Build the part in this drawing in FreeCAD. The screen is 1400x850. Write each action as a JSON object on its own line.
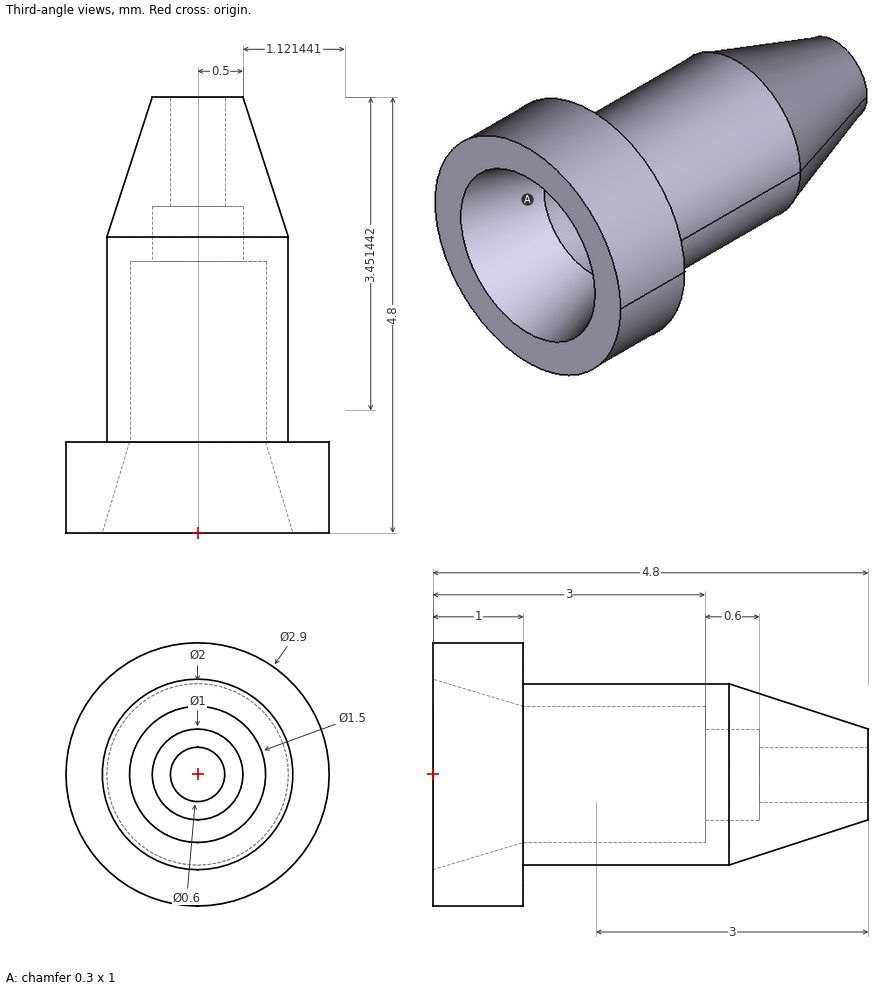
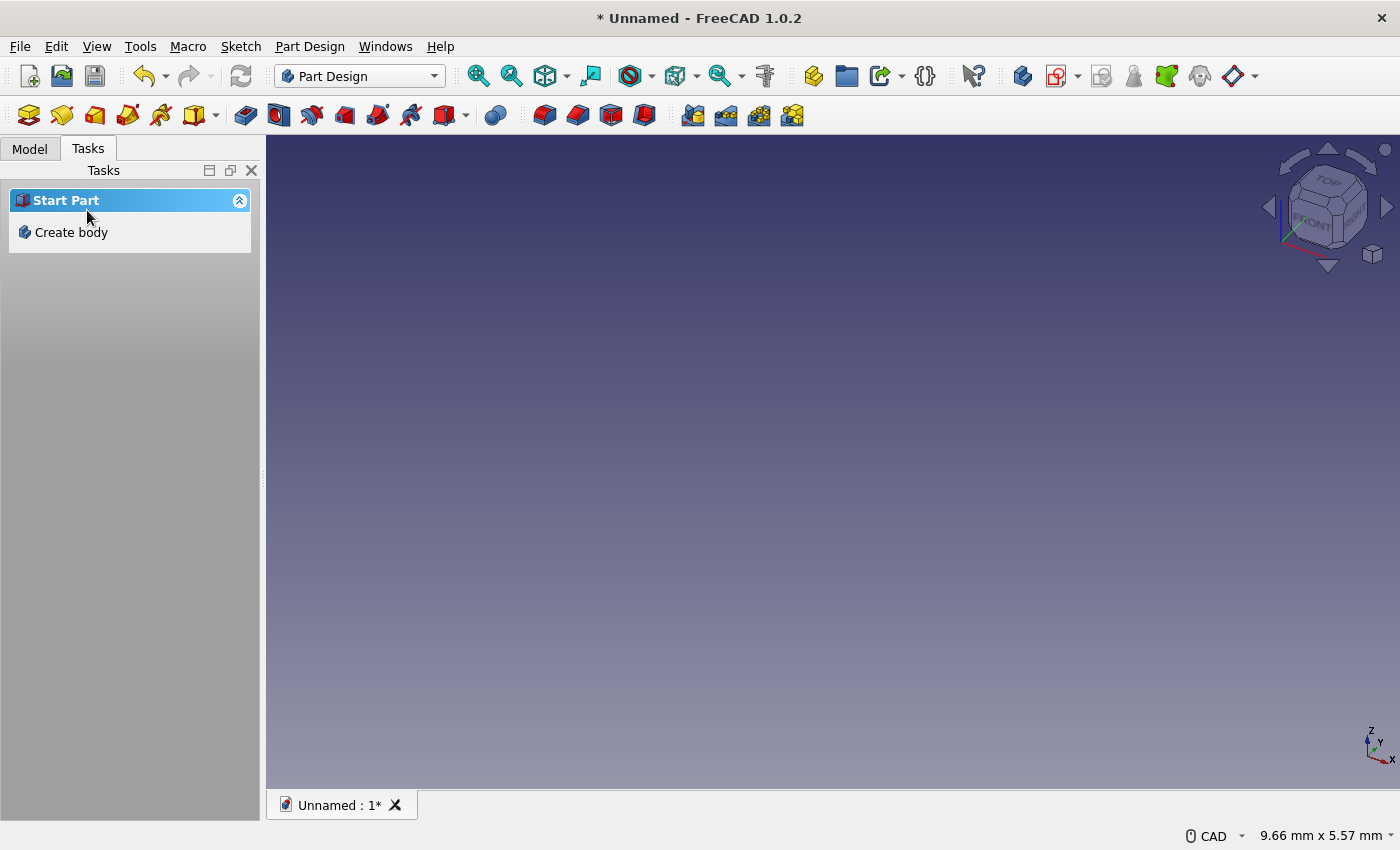
{"action": "left_click", "coordinate": [479, 76]}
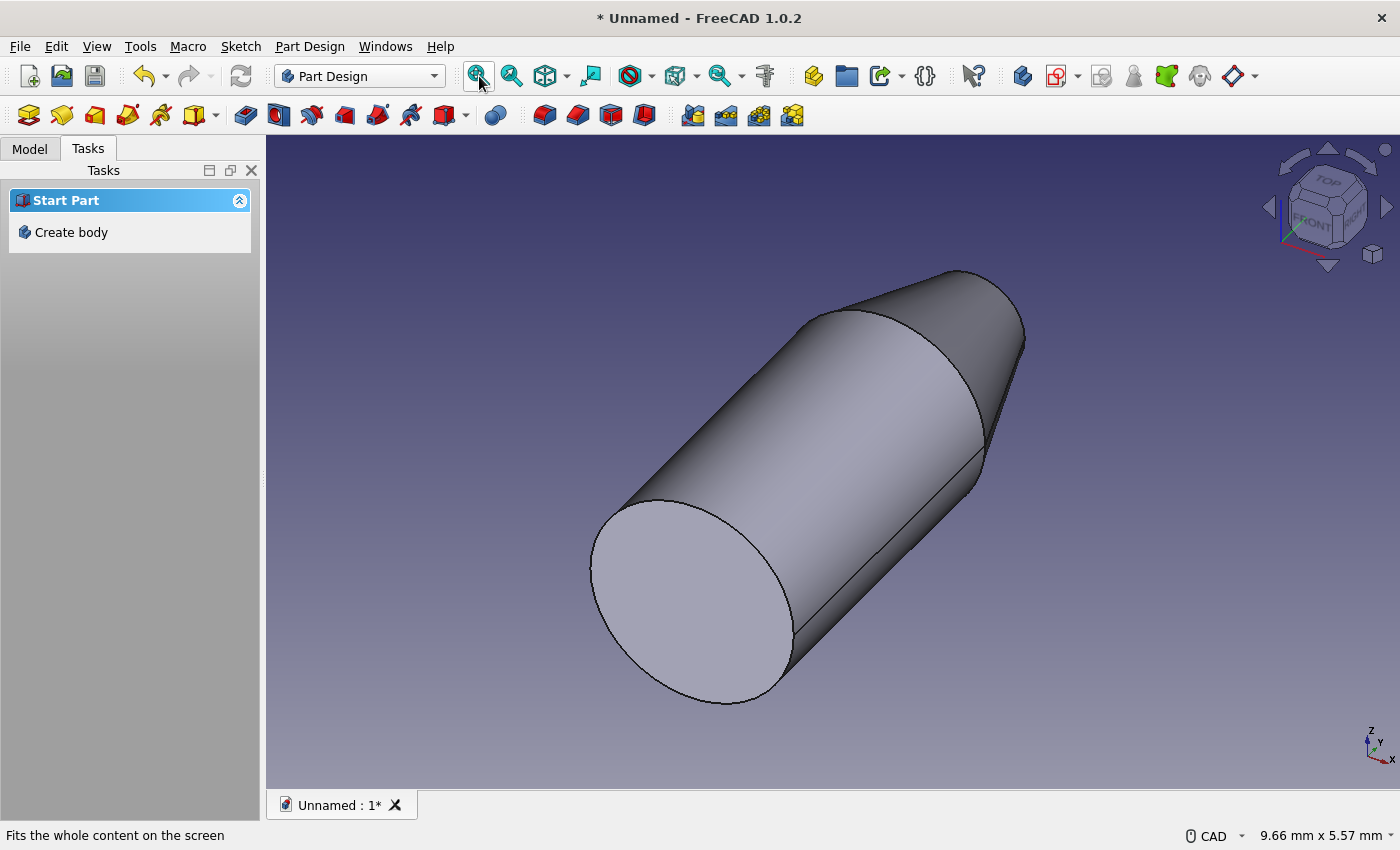
{"action": "left_click", "coordinate": [692, 601]}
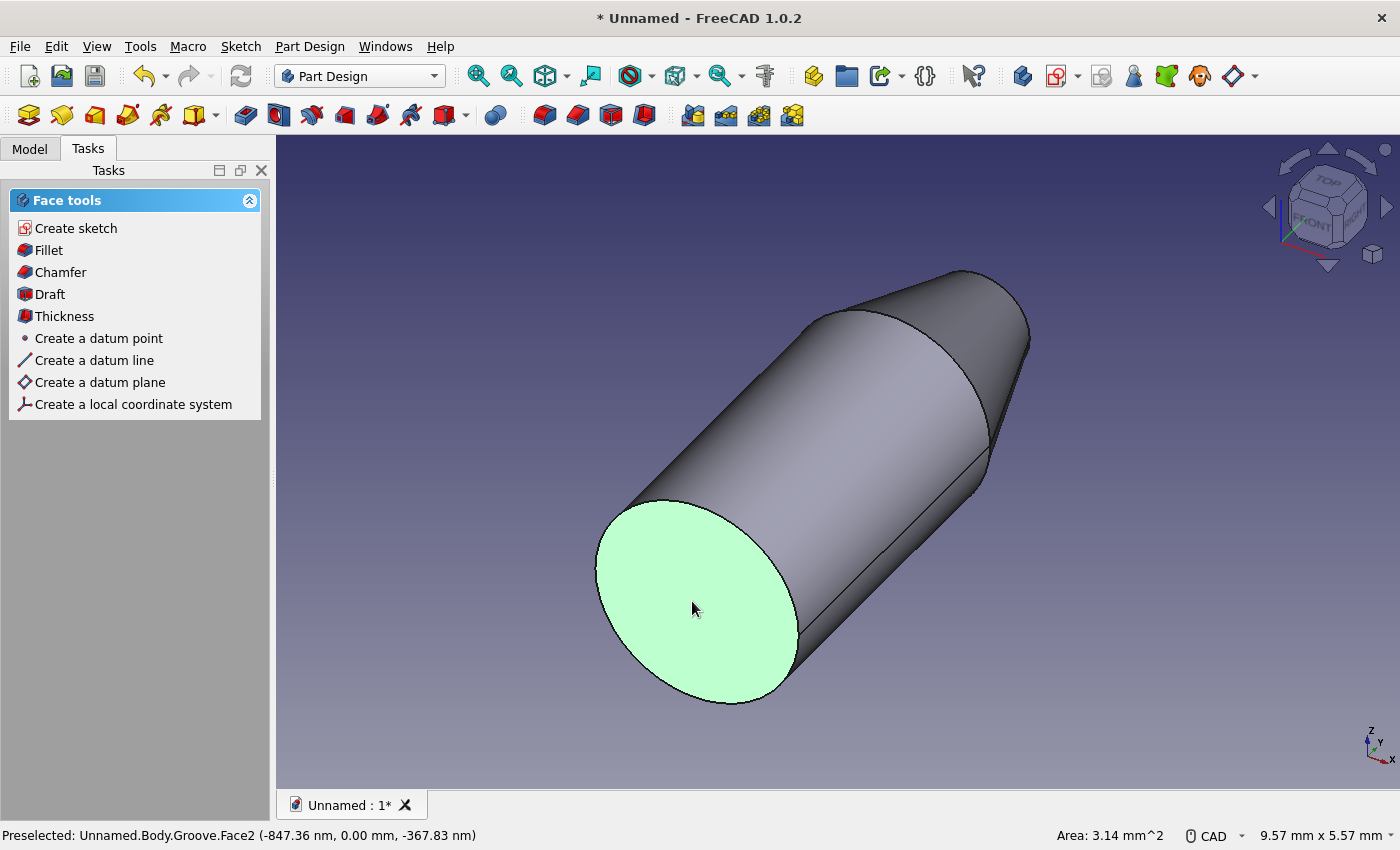
{"action": "left_click", "coordinate": [1056, 76]}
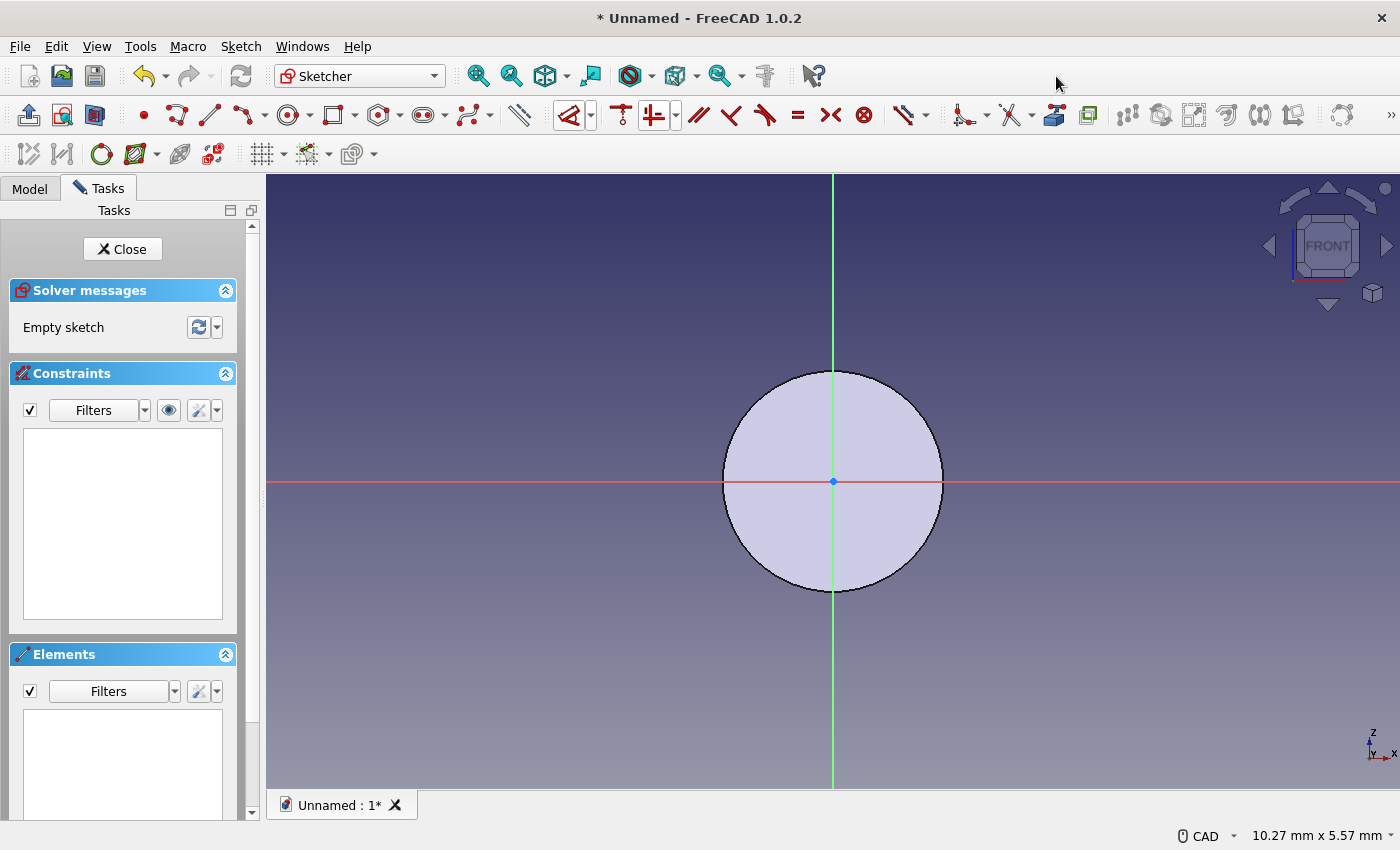
{"action": "scroll", "coordinate": [889, 482], "scroll_direction": "up", "scroll_amount": 4}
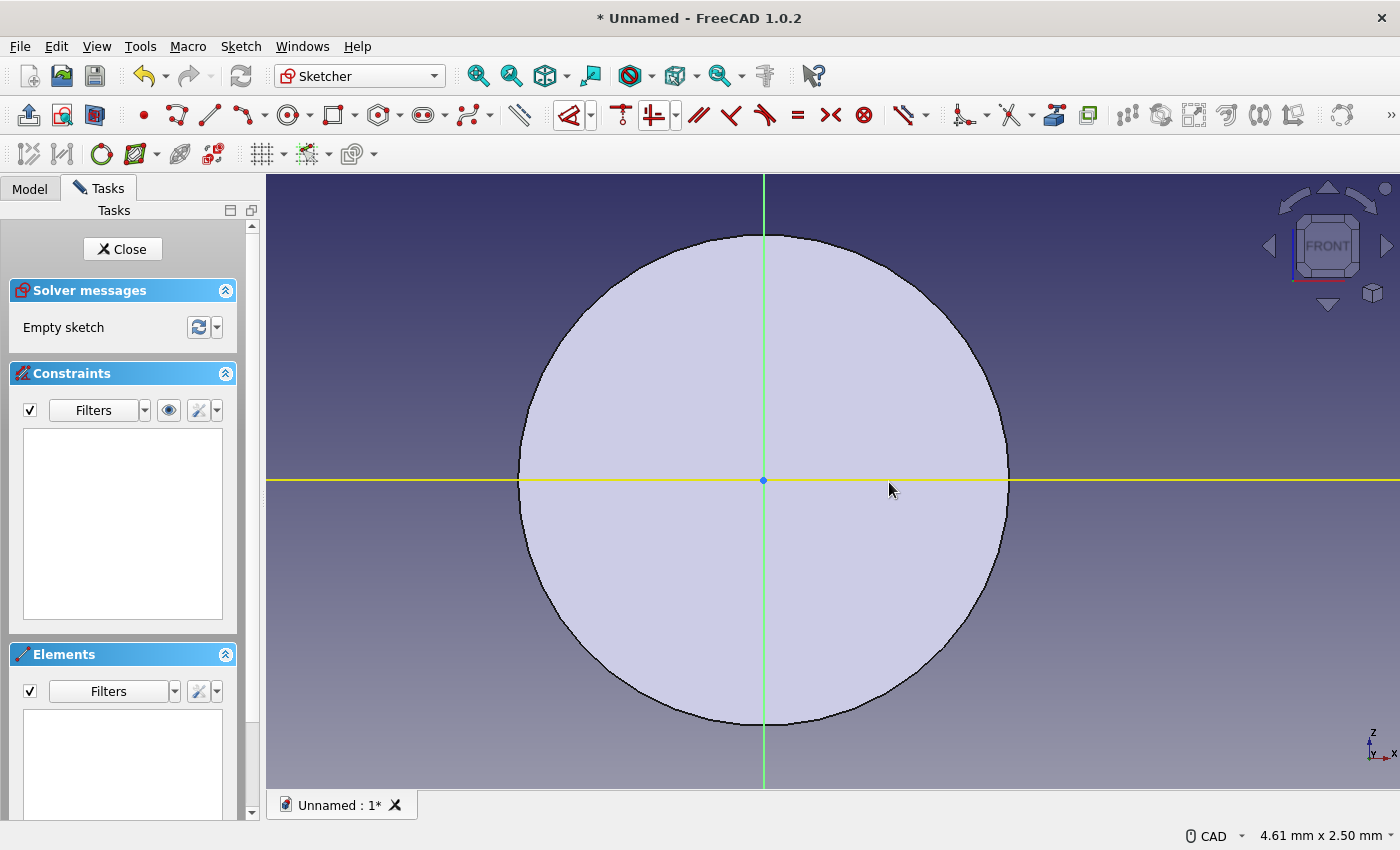
{"action": "left_click", "coordinate": [288, 116]}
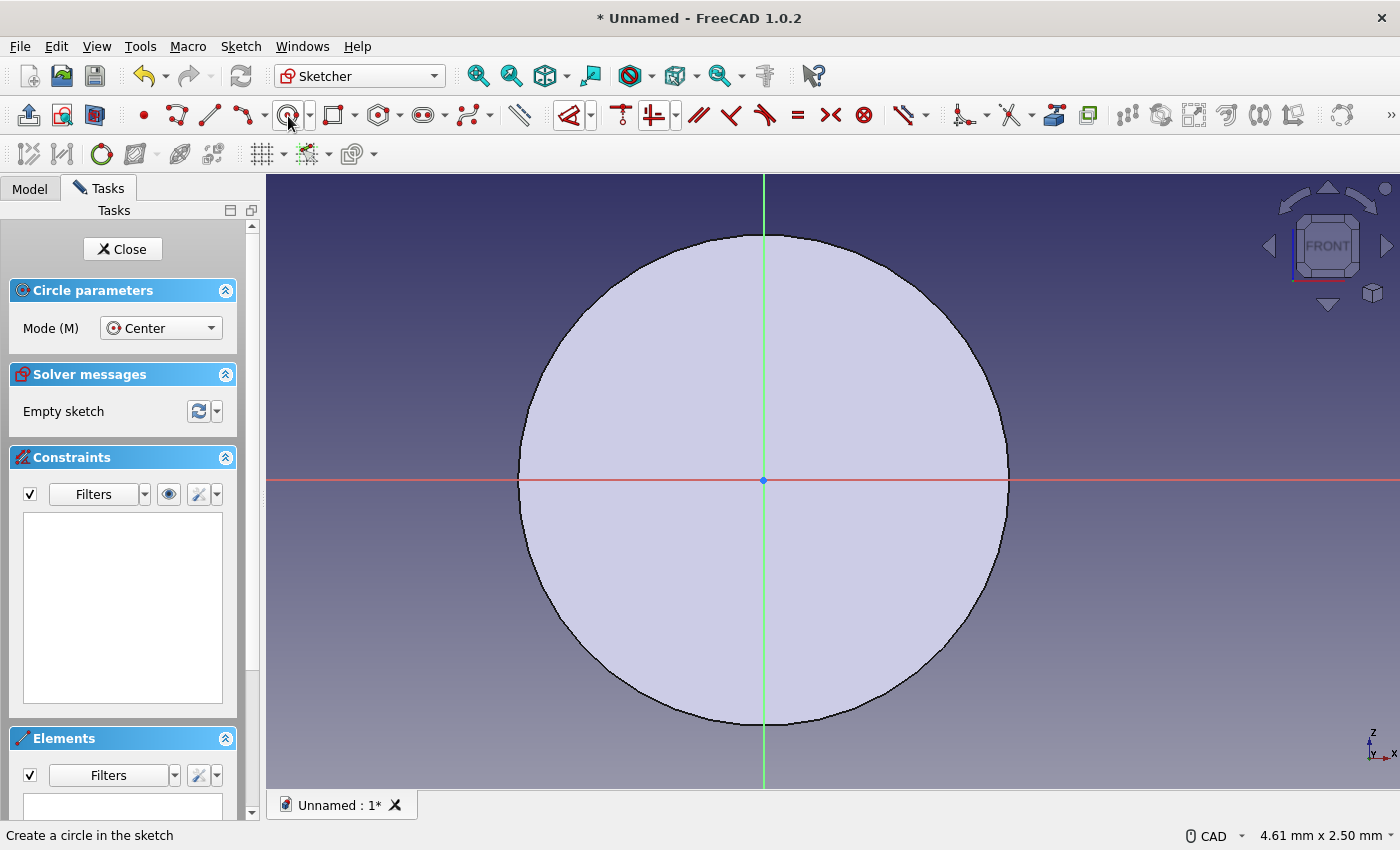
{"action": "left_click", "coordinate": [764, 480]}
{"action": "left_click", "coordinate": [894, 350]}
{"action": "key", "text": "Escape"}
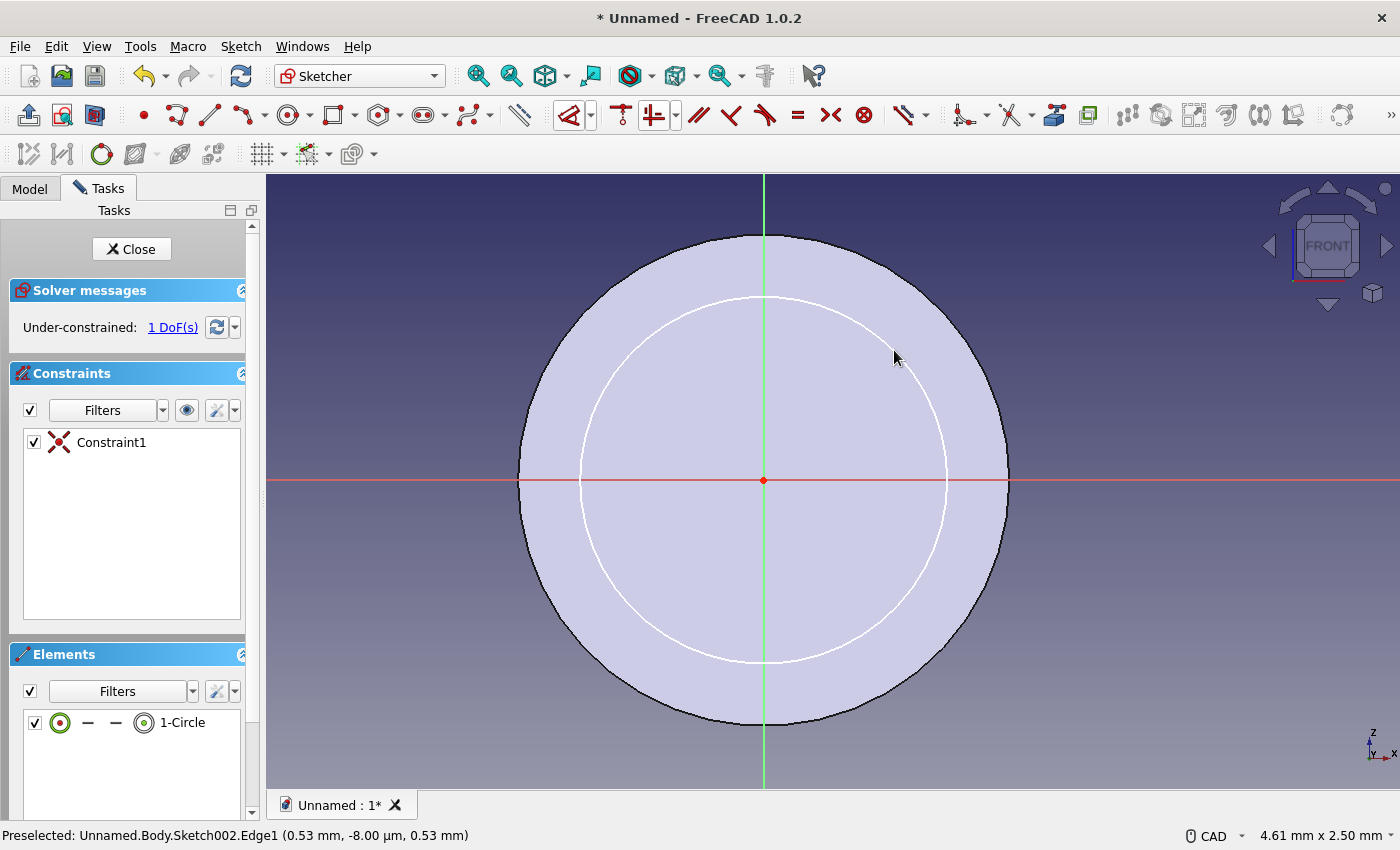
{"action": "left_click", "coordinate": [893, 350]}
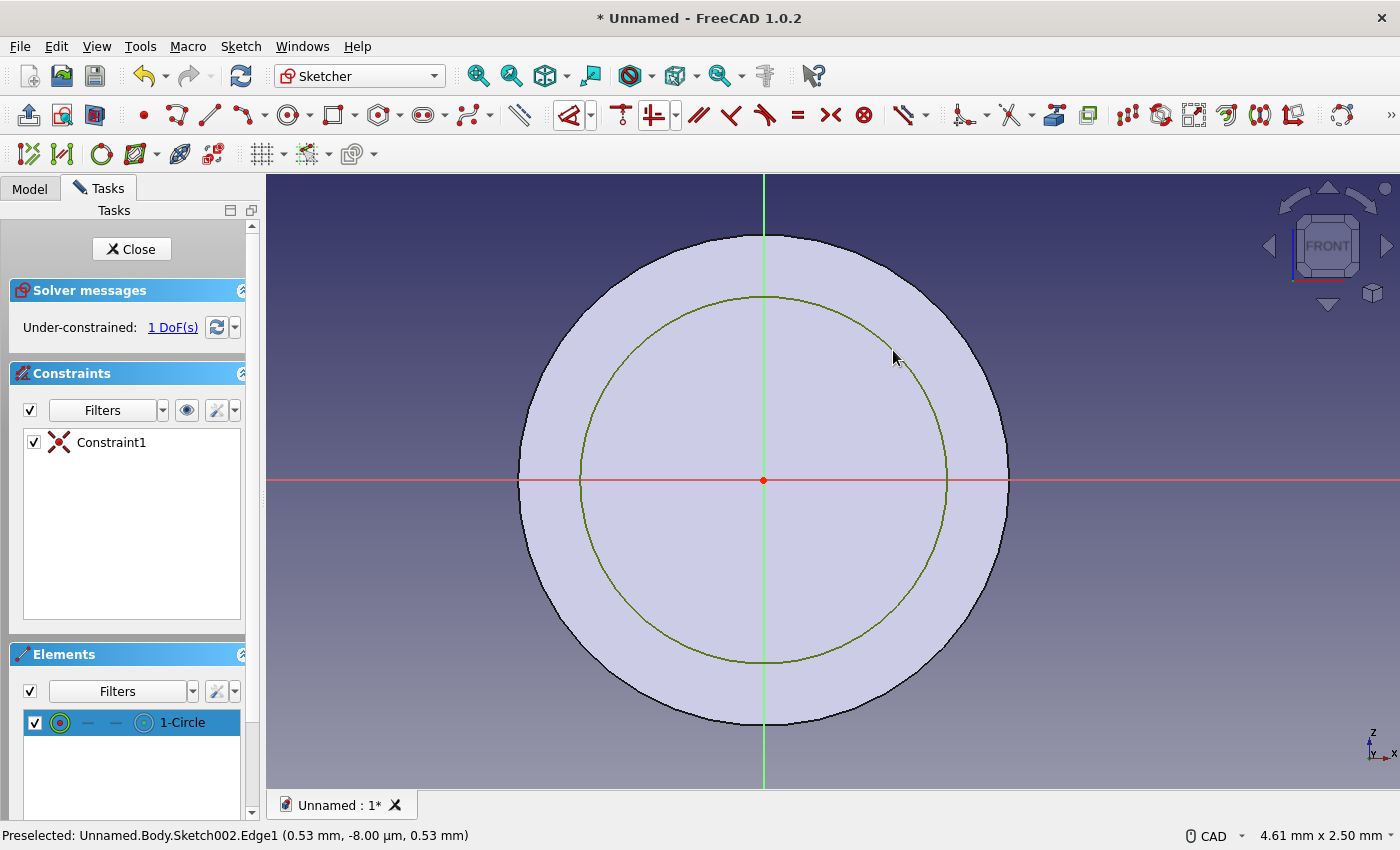
{"action": "key", "text": "k o"}